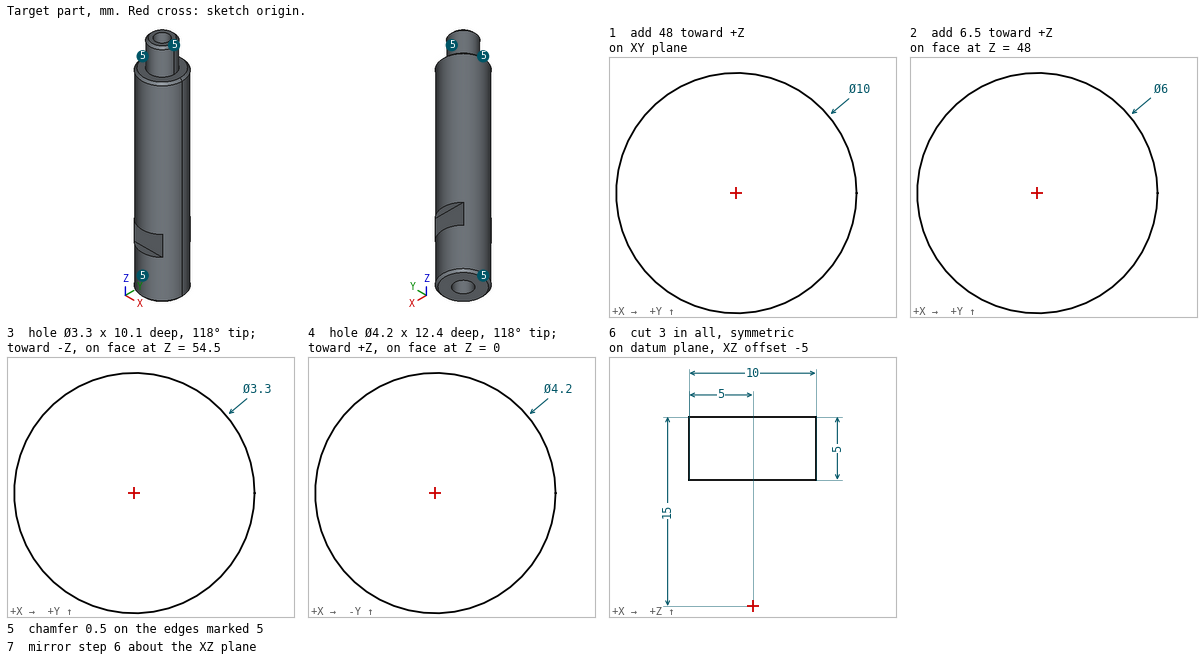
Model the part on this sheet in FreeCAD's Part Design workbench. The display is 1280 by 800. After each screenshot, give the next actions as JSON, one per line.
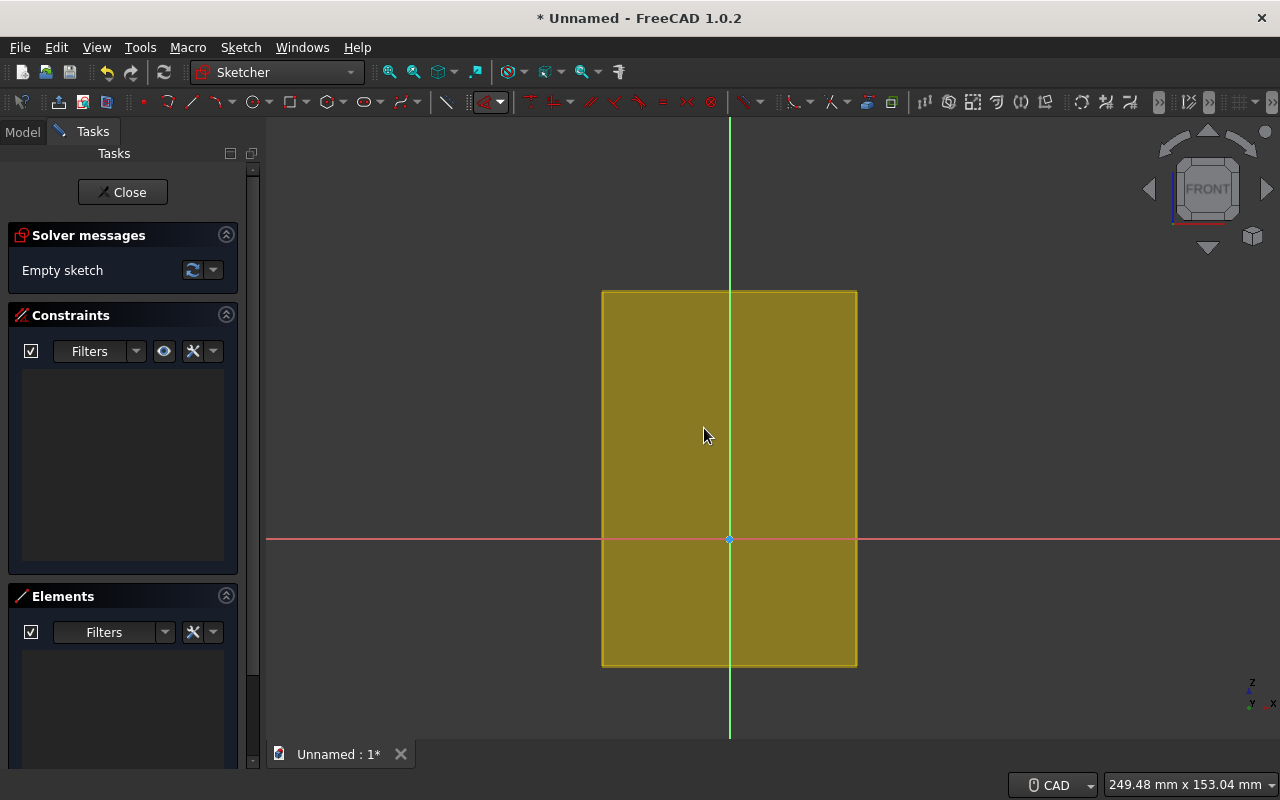
{"action": "scroll", "coordinate": [735, 525], "scroll_direction": "up", "scroll_amount": 9}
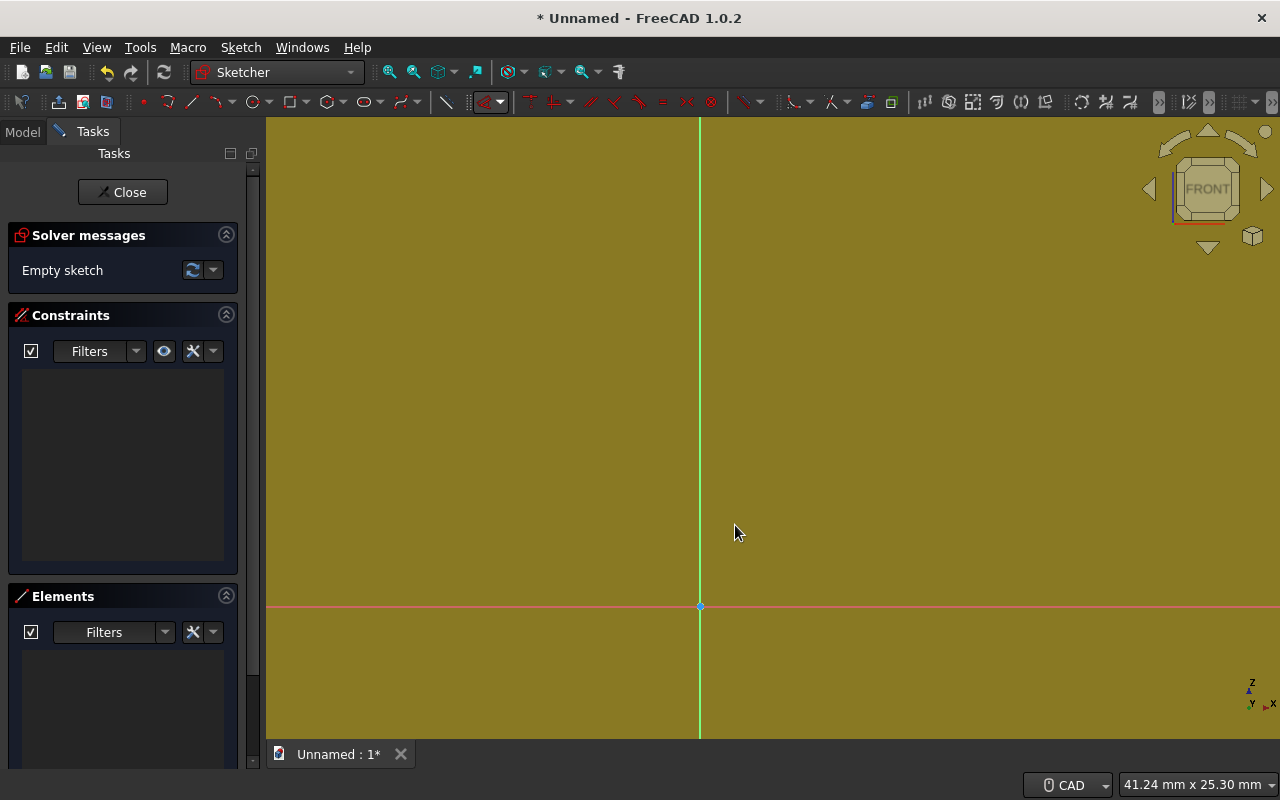
{"action": "left_click", "coordinate": [290, 102]}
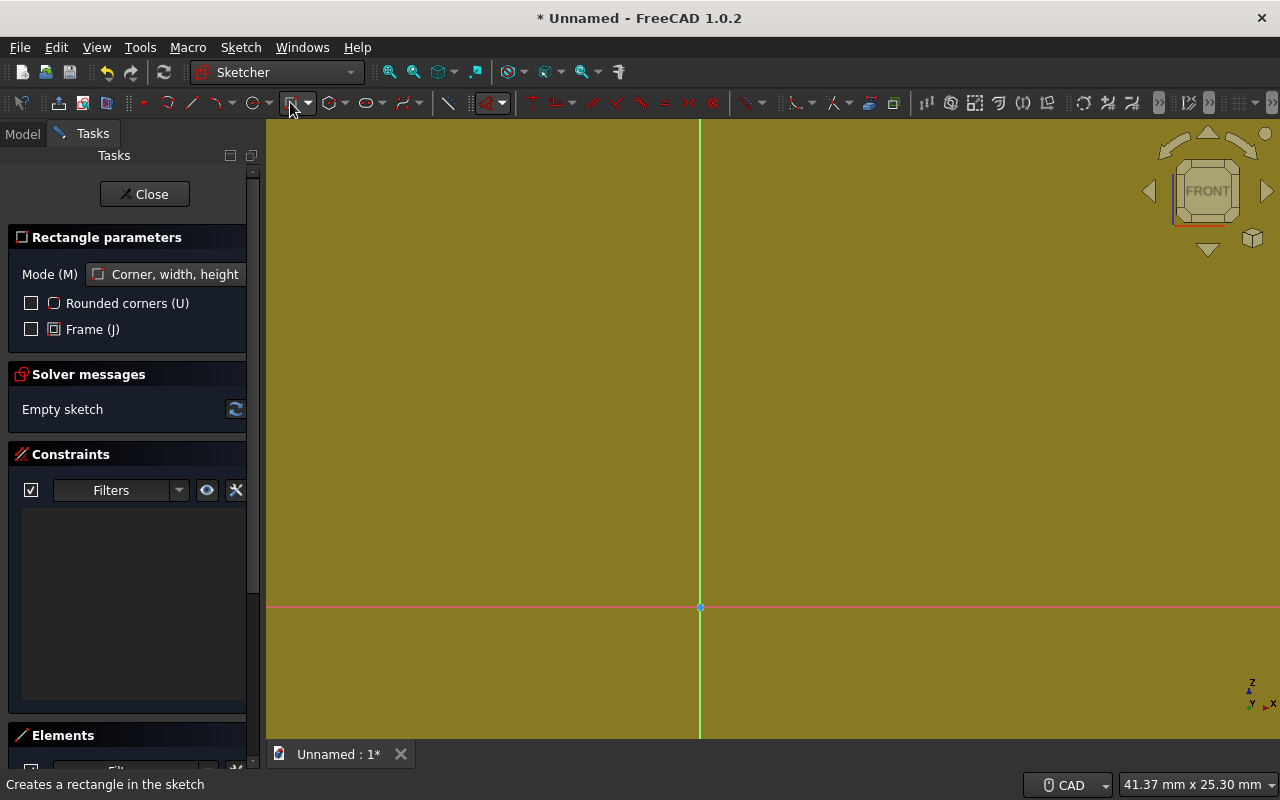
{"action": "left_click", "coordinate": [578, 240]}
{"action": "mouse_move", "coordinate": [823, 362]}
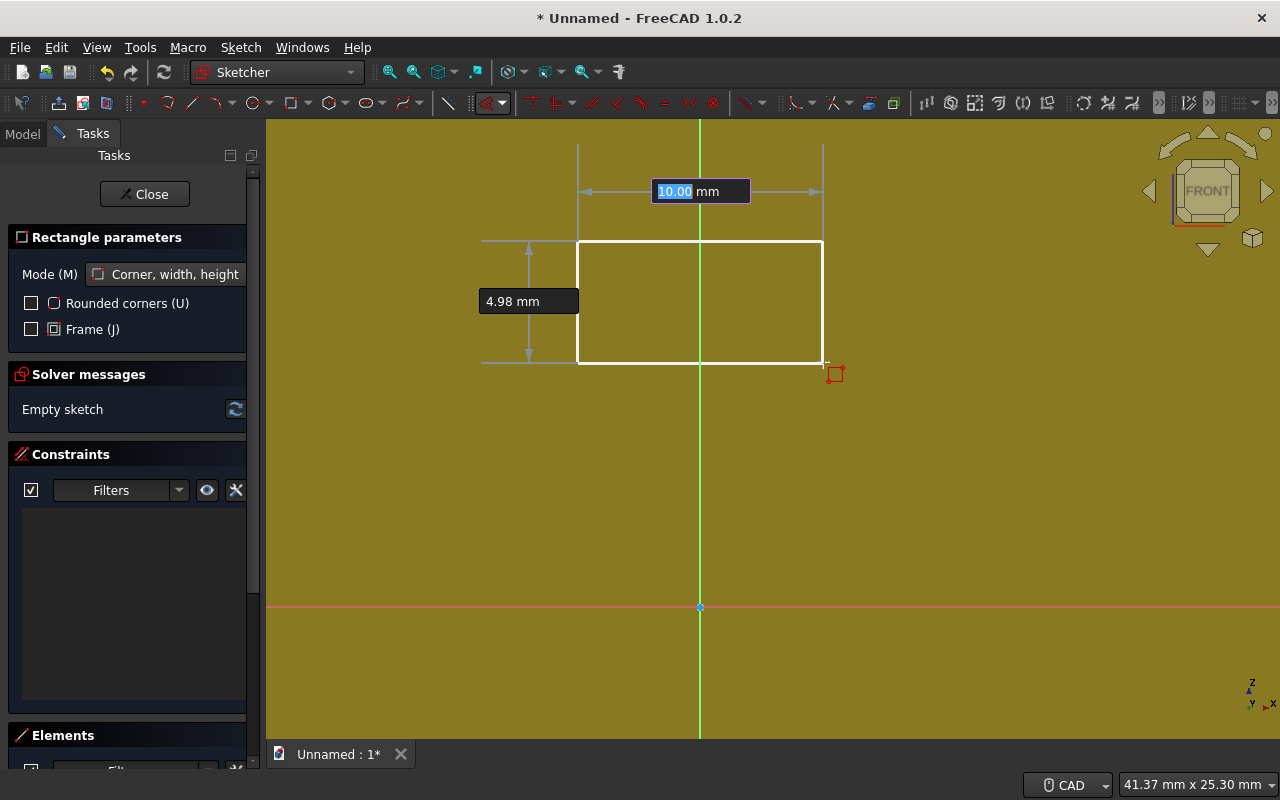
{"action": "type", "text": "10"}
{"action": "key", "text": "Tab"}
{"action": "type", "text": "5"}
{"action": "key", "text": "Return"}
{"action": "key", "text": "Escape"}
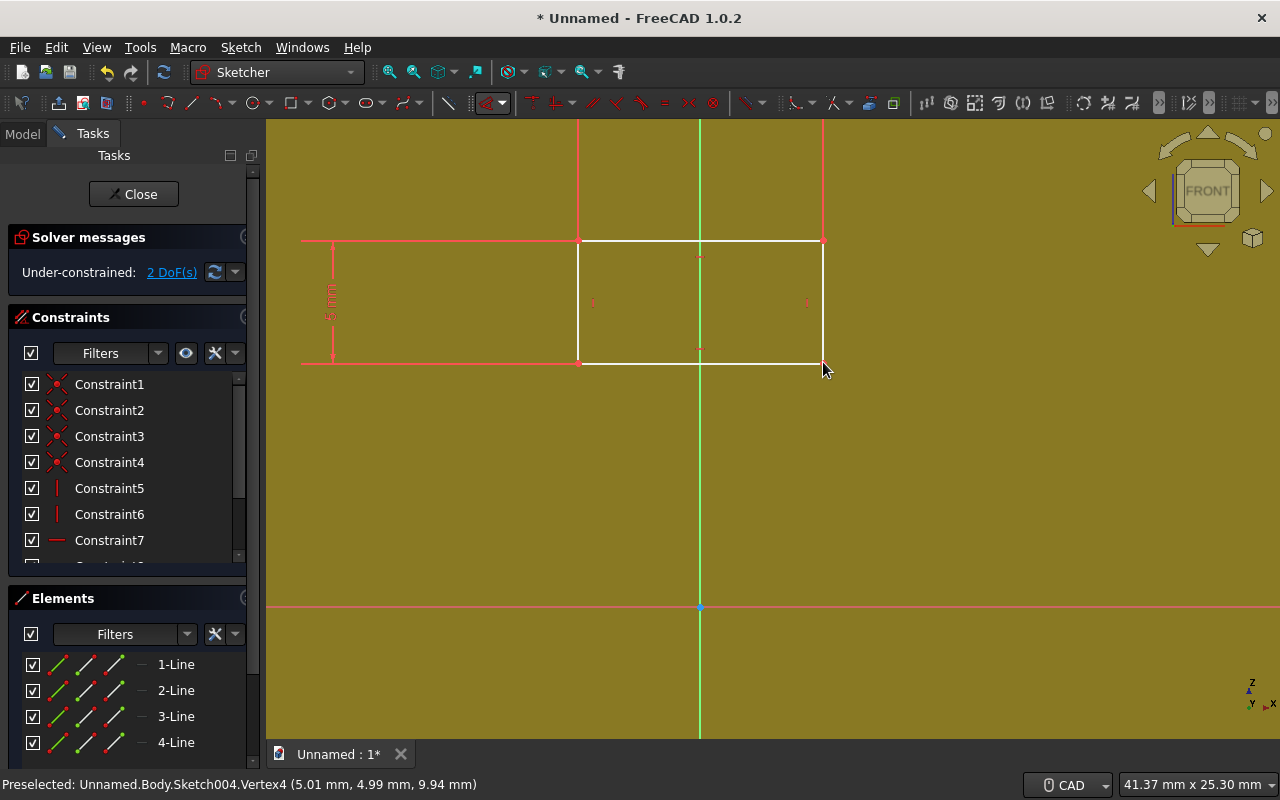
{"action": "left_click", "coordinate": [486, 104]}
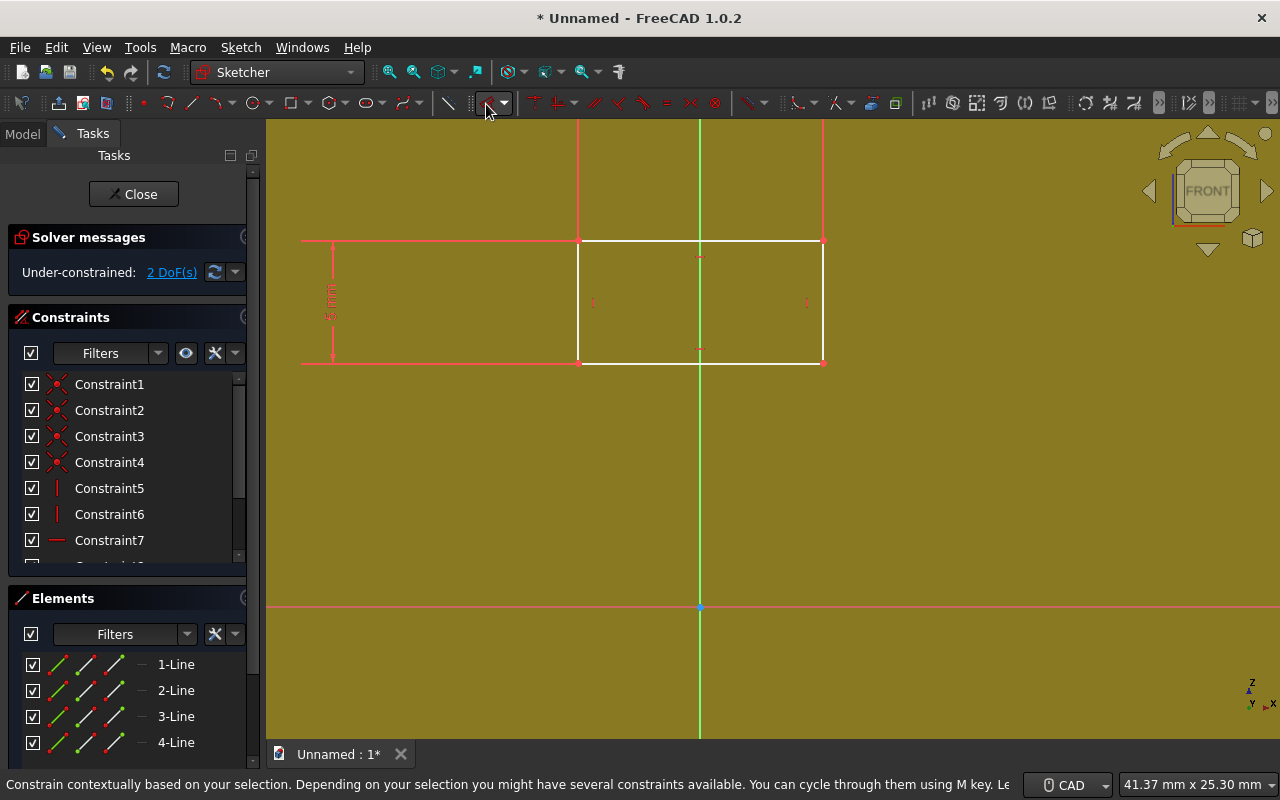
{"action": "left_click", "coordinate": [578, 241]}
{"action": "left_click", "coordinate": [639, 641]}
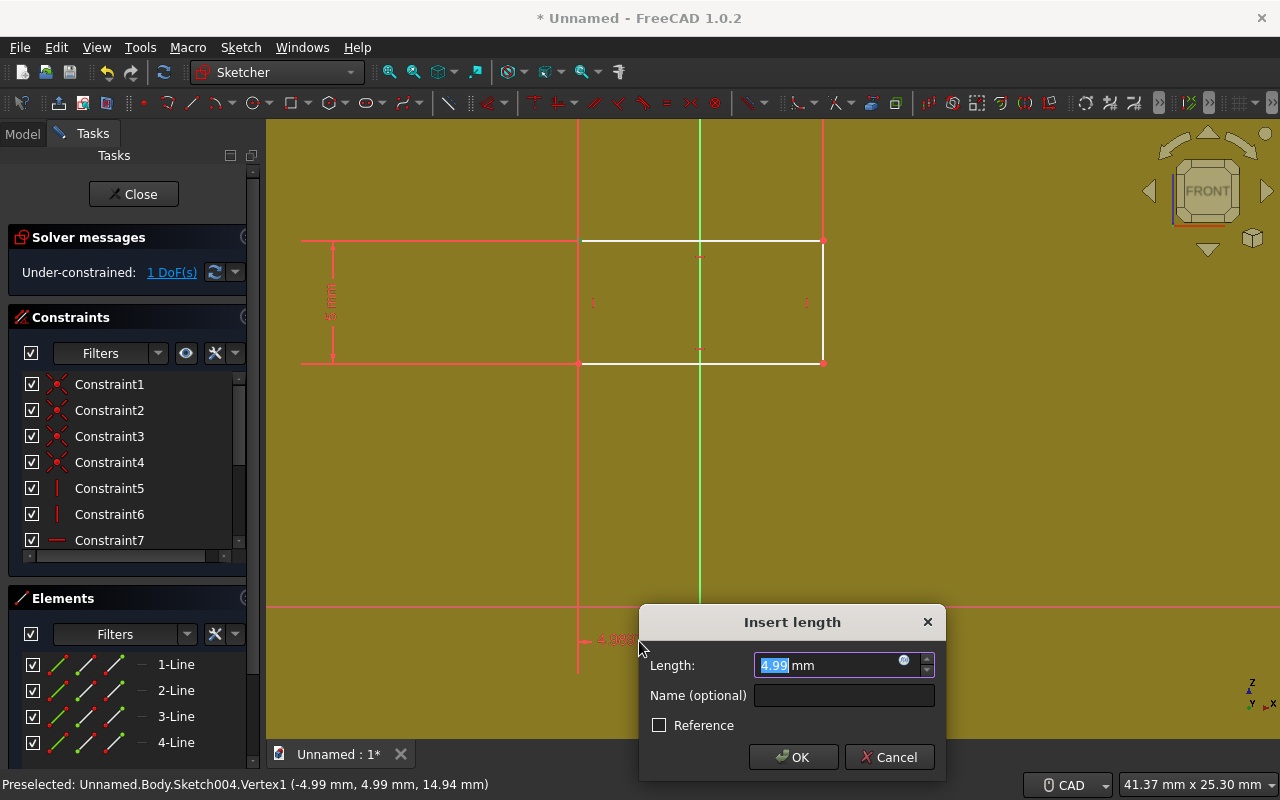
{"action": "type", "text": "5"}
{"action": "key", "text": "Return"}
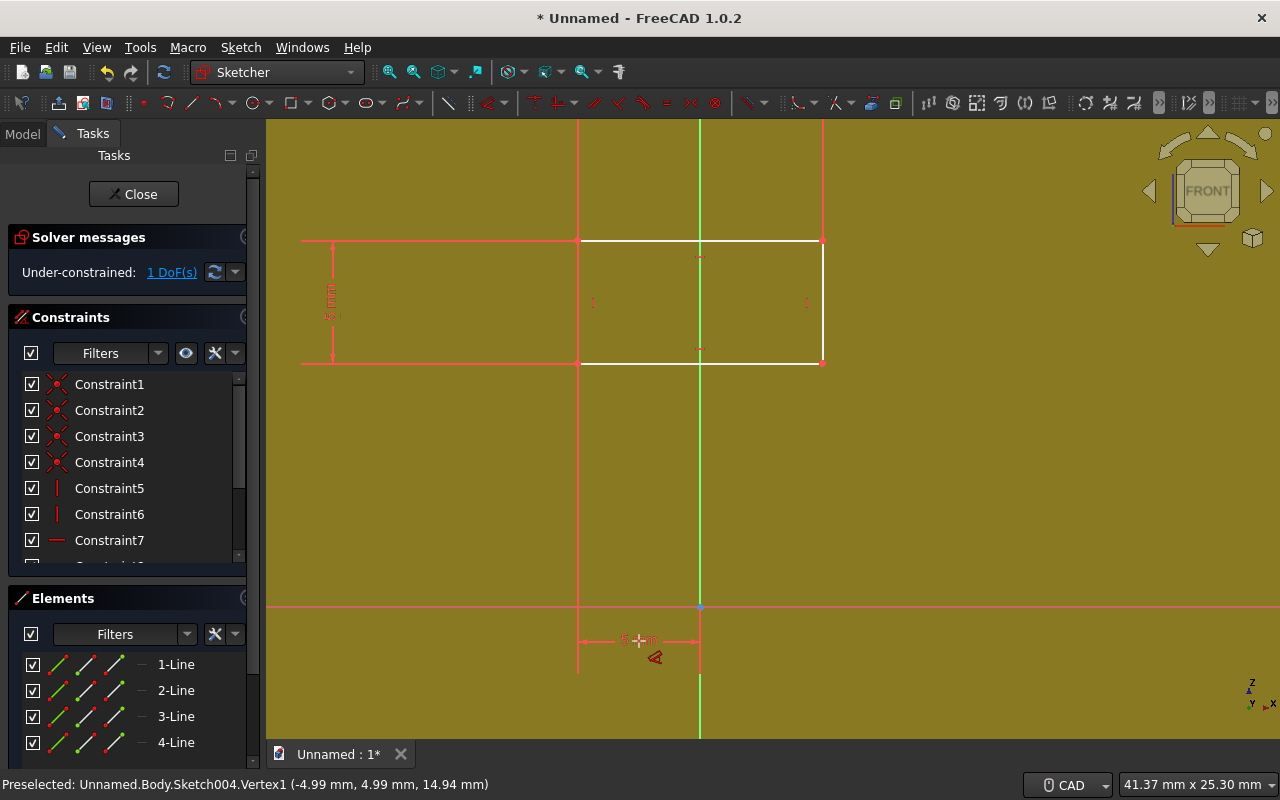
{"action": "left_click", "coordinate": [578, 241]}
{"action": "left_click", "coordinate": [544, 424]}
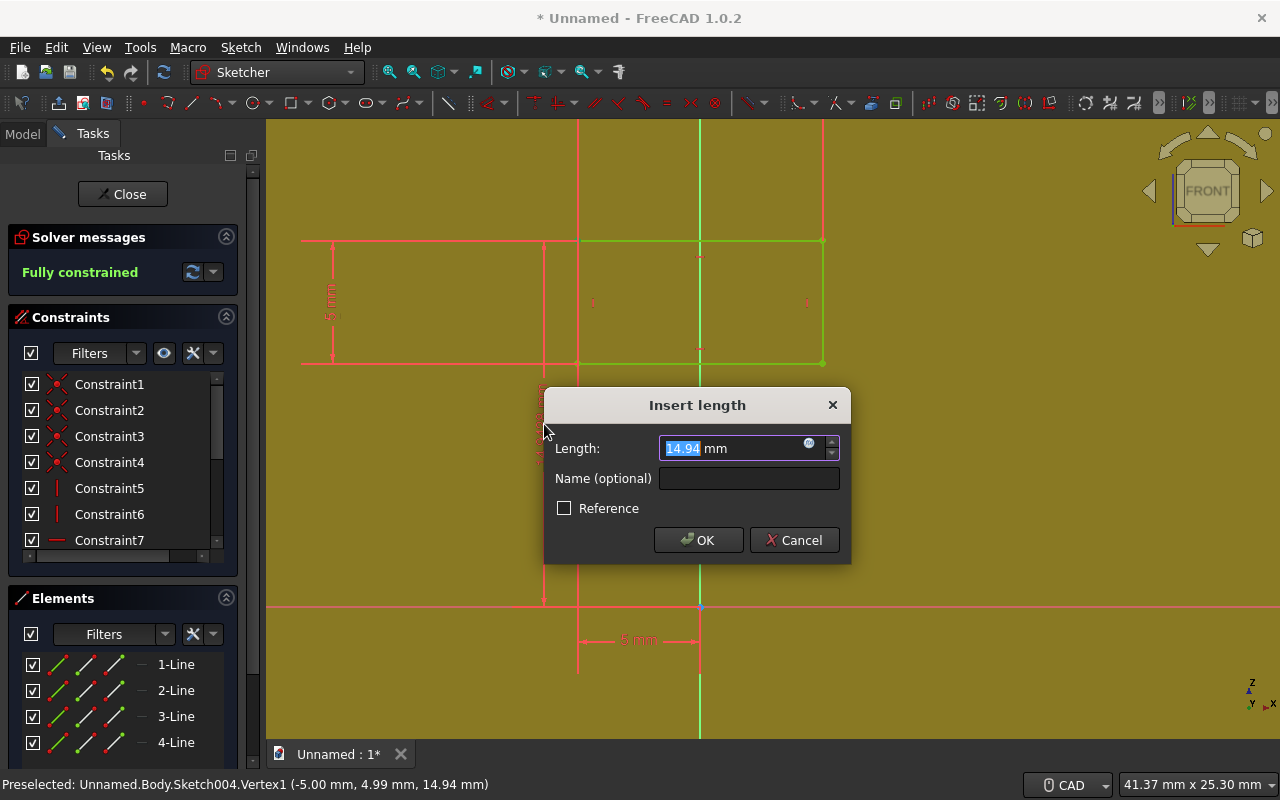
{"action": "type", "text": "15"}
{"action": "key", "text": "Return"}
{"action": "key", "text": "Escape"}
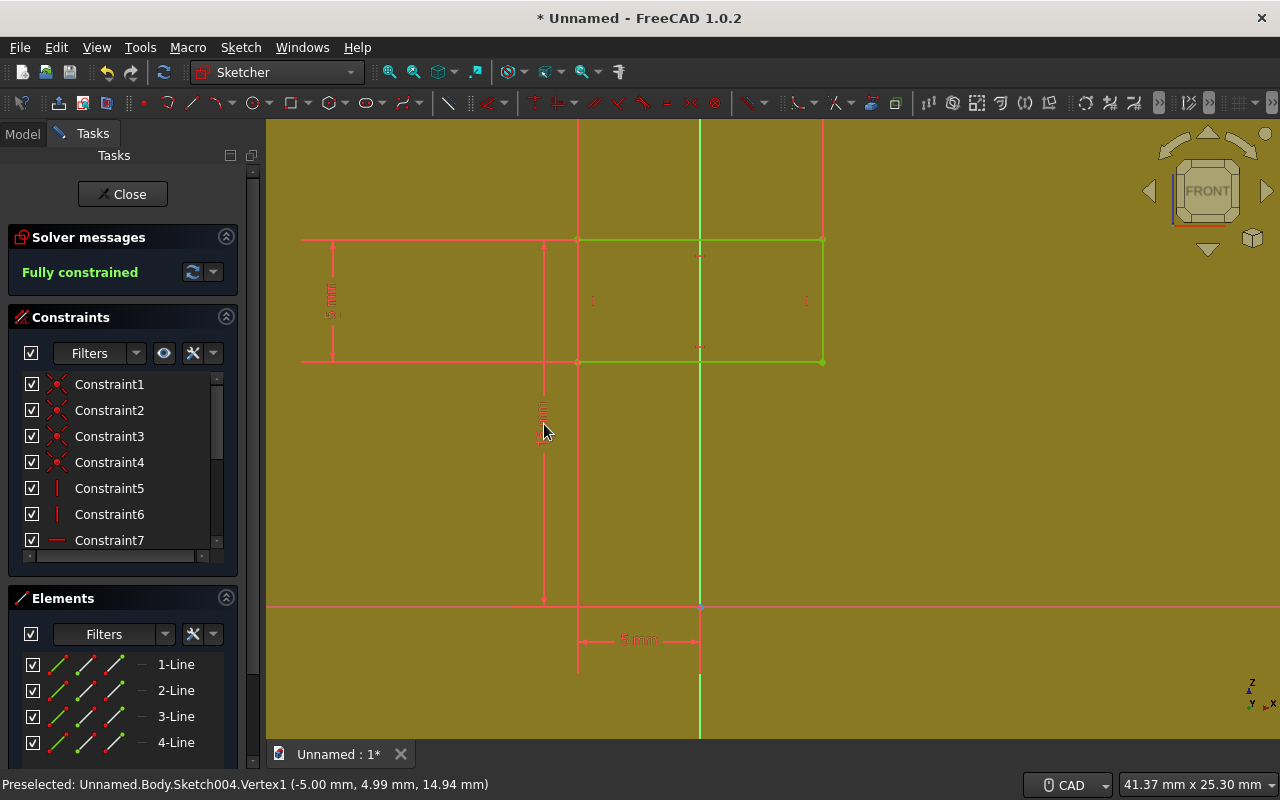
{"action": "left_click", "coordinate": [123, 194]}